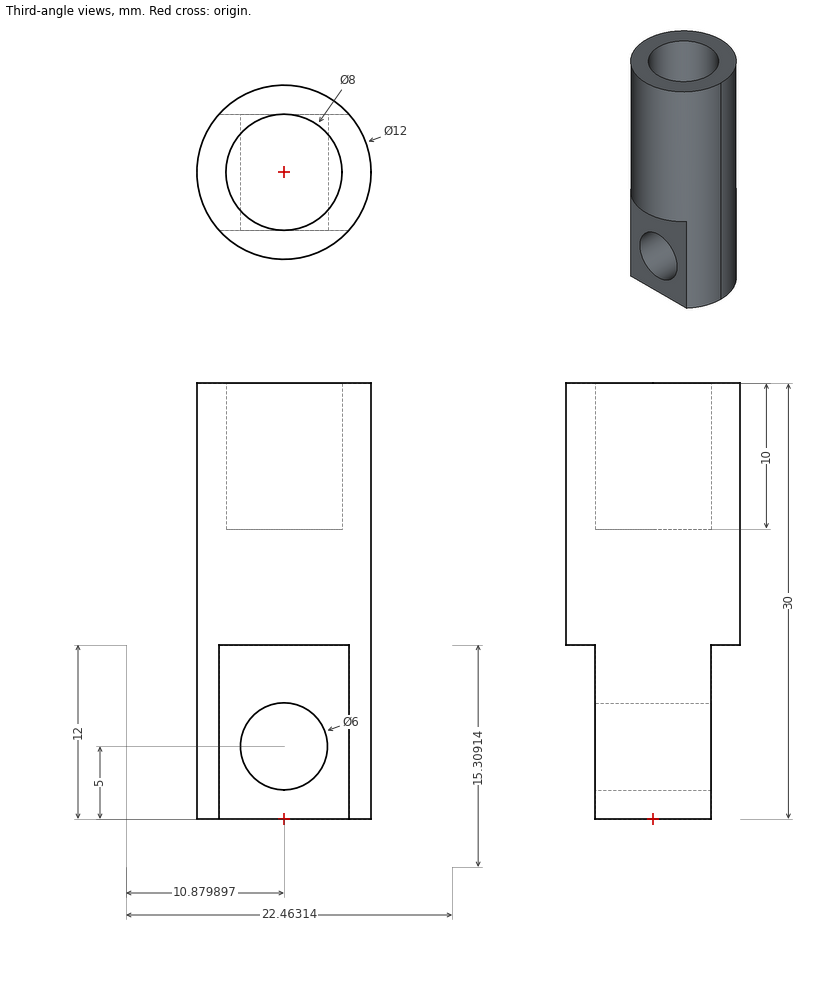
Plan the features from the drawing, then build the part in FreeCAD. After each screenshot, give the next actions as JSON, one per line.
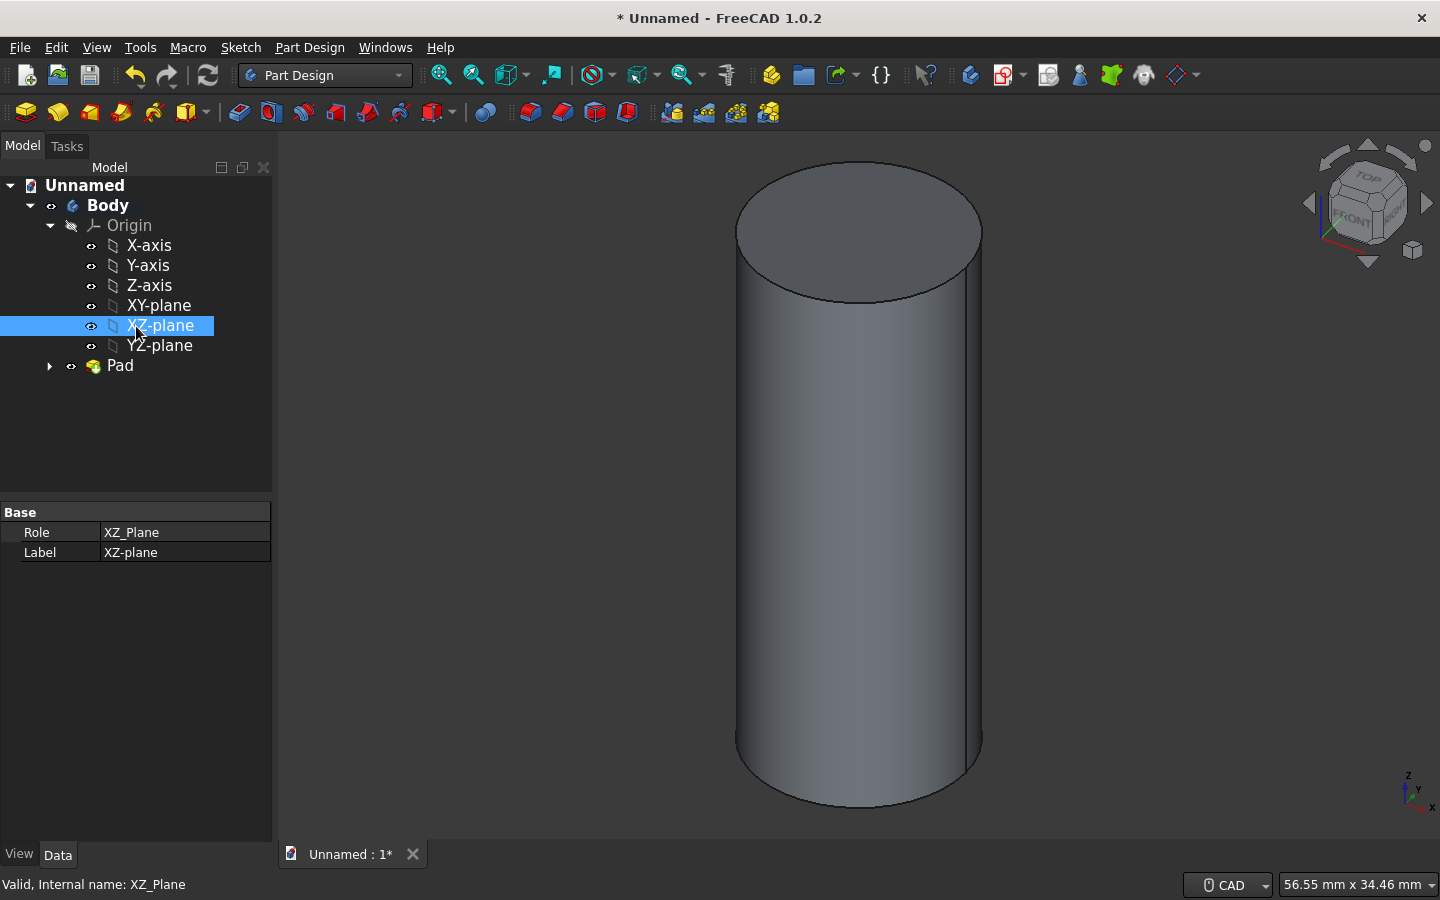
{"action": "left_click", "coordinate": [1176, 76]}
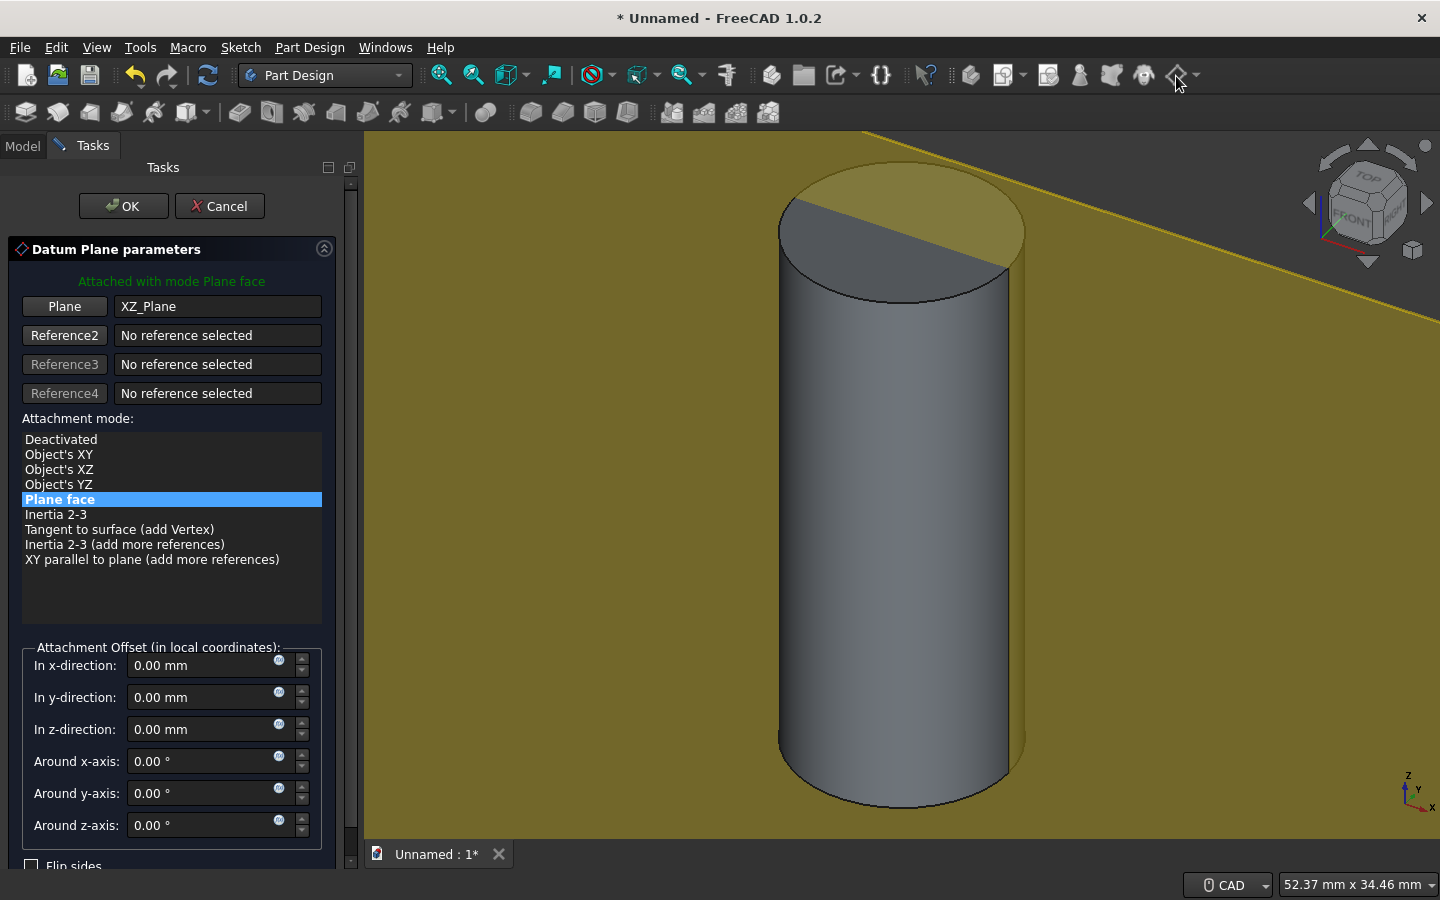
{"action": "triple_click", "coordinate": [210, 729]}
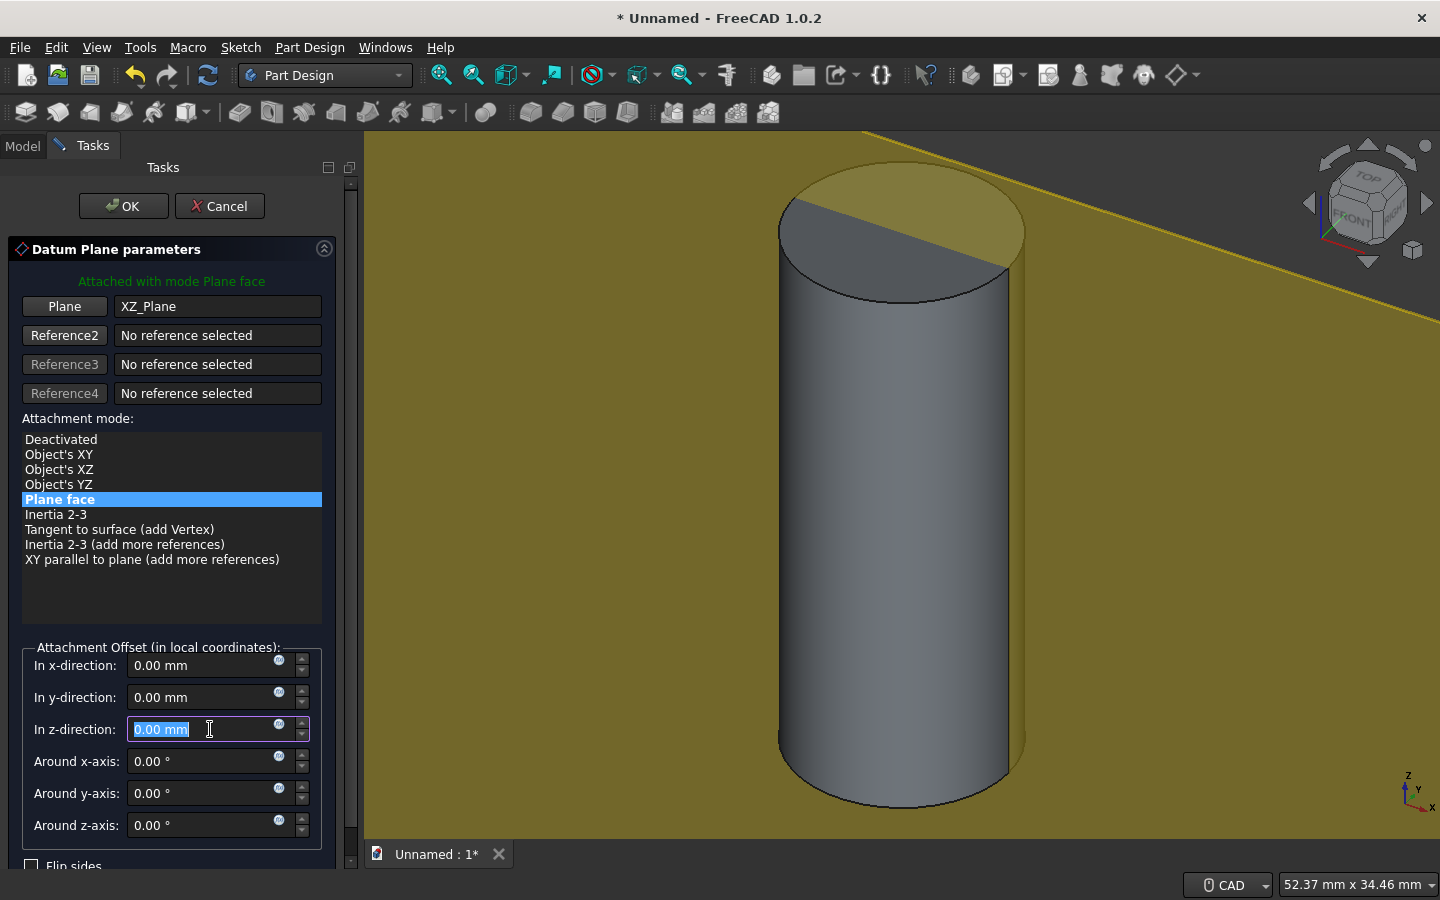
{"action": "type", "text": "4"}
{"action": "key", "text": "Tab"}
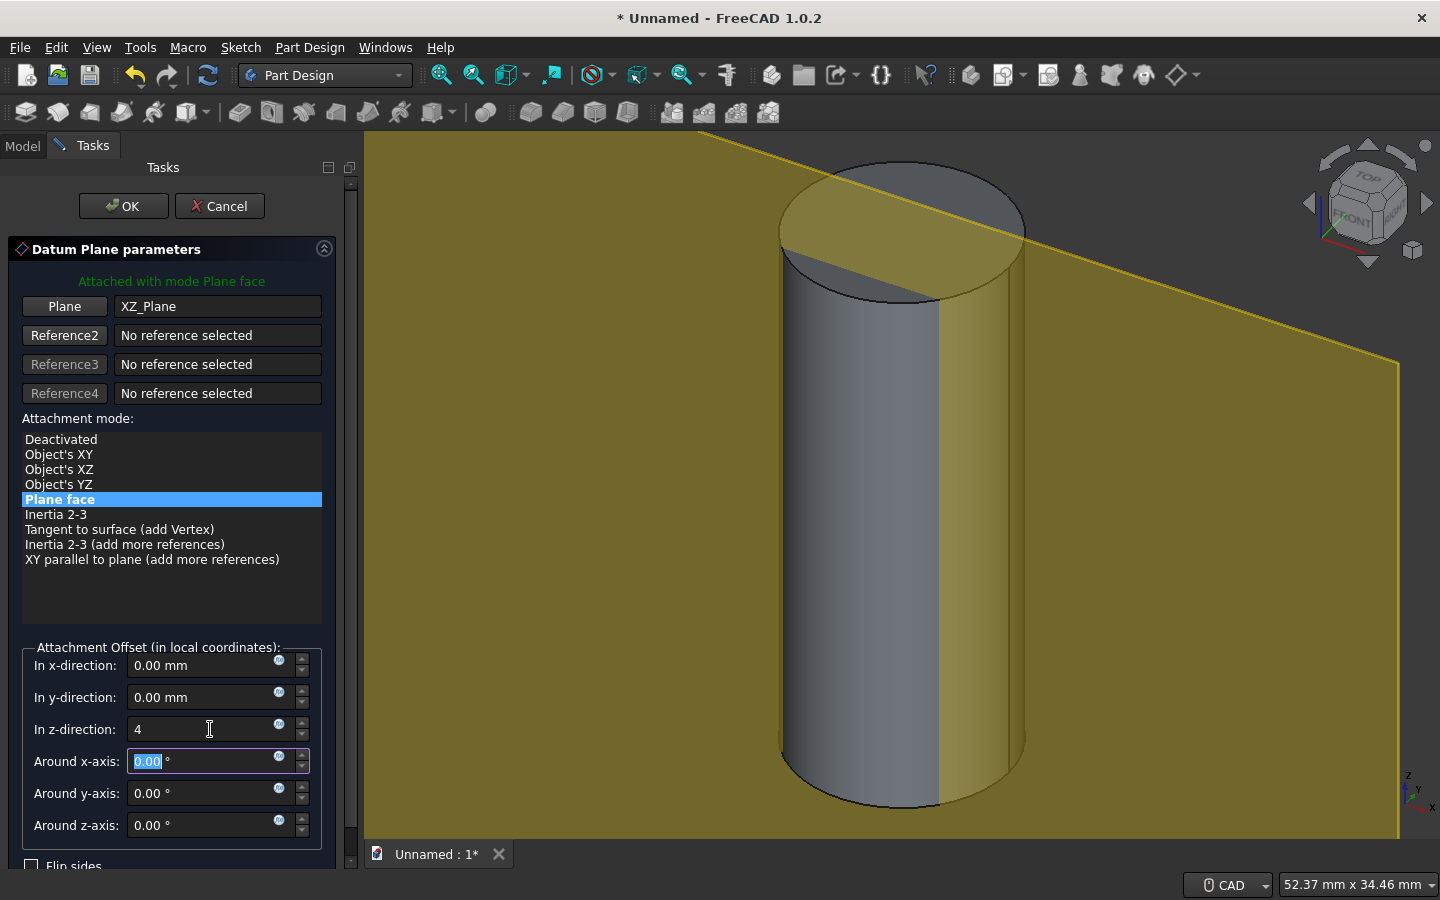
{"action": "left_click", "coordinate": [124, 206]}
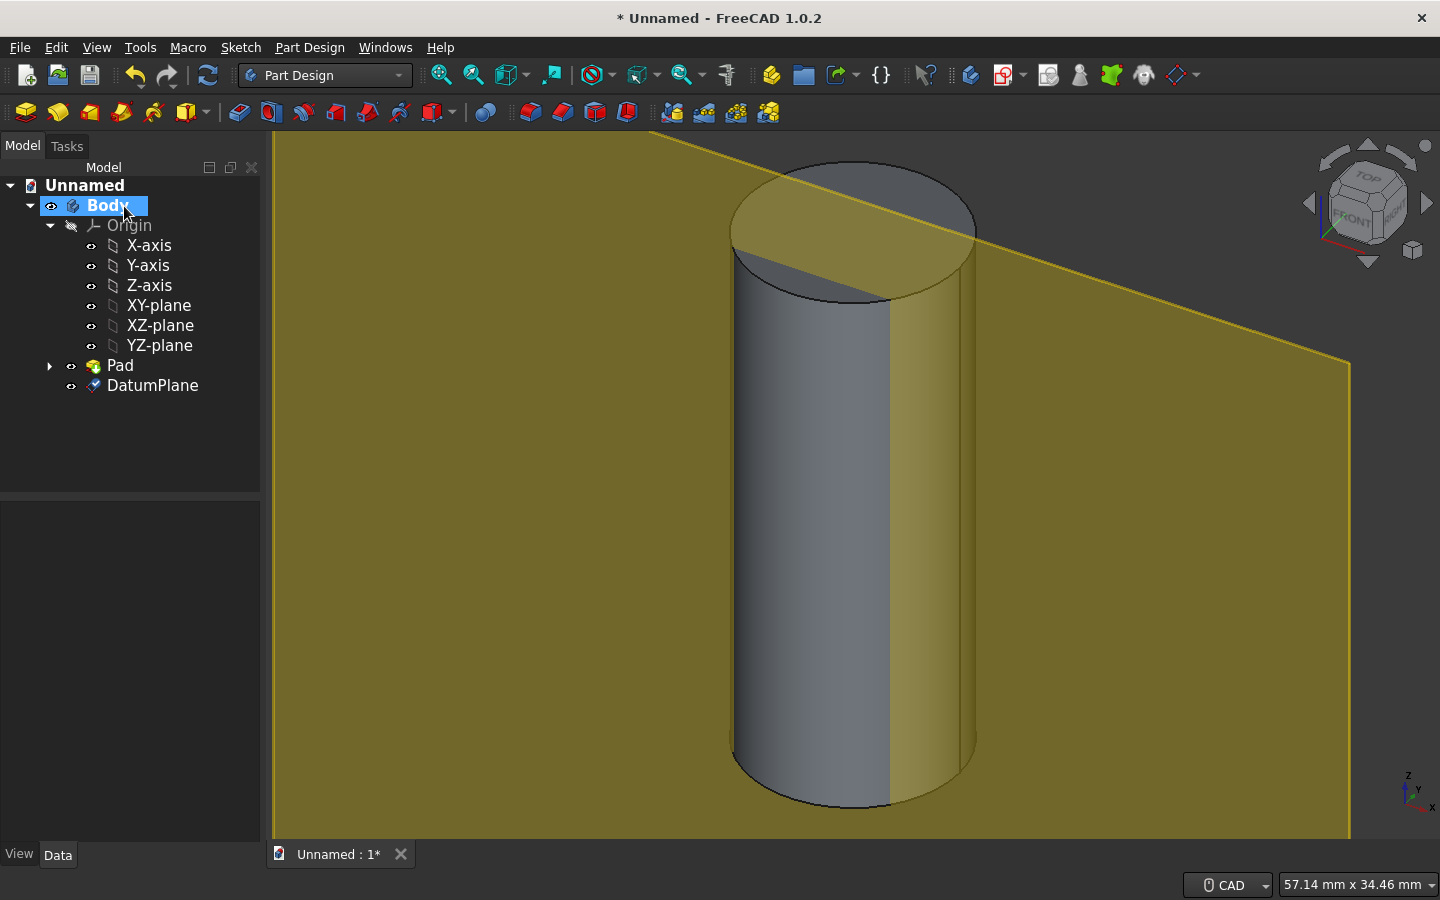
{"action": "left_click", "coordinate": [116, 386]}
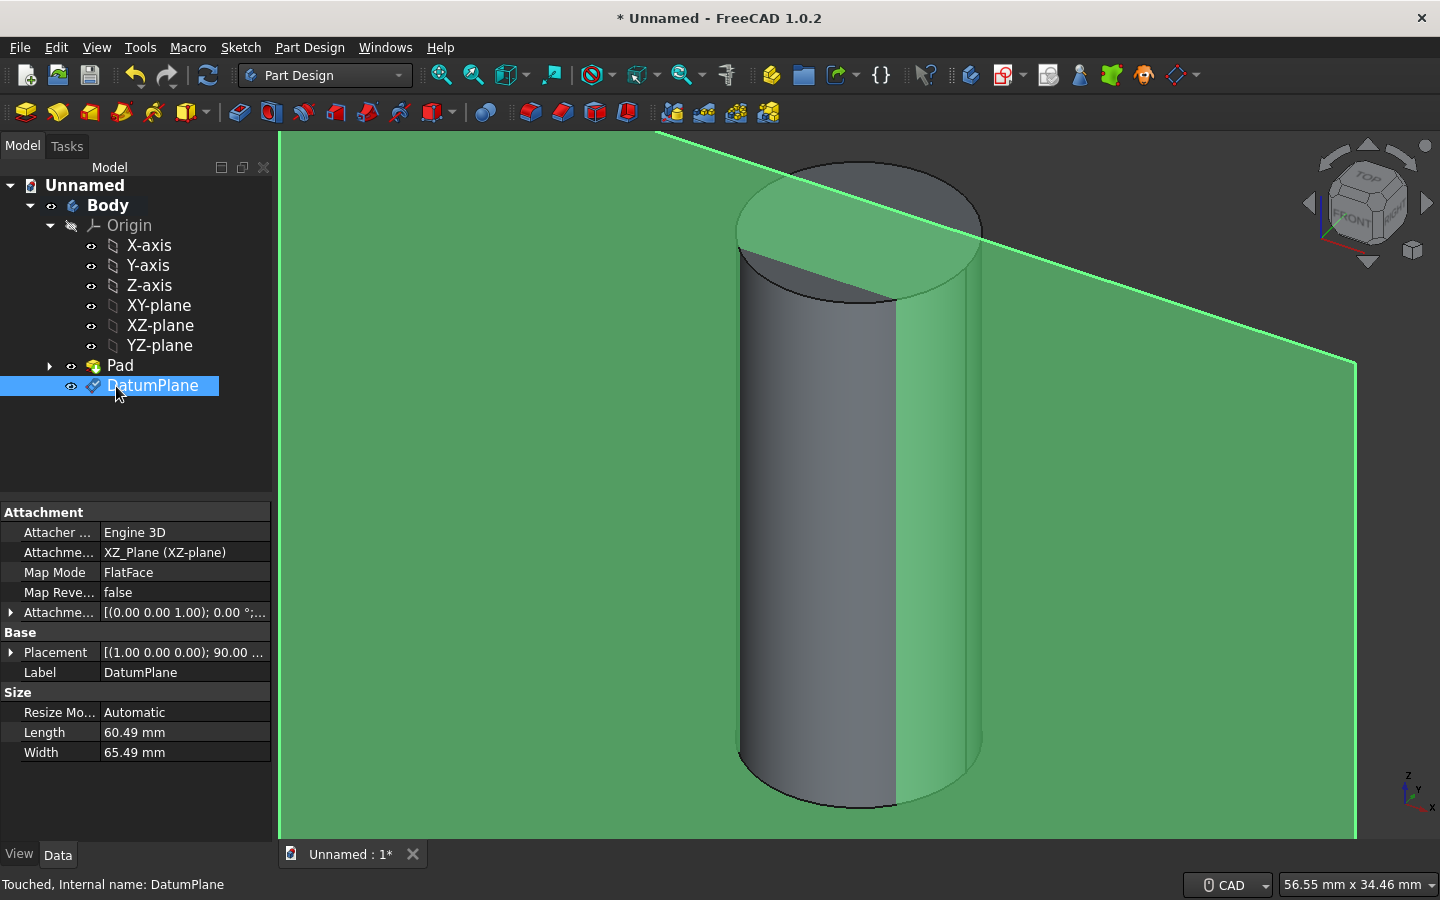
{"action": "left_click", "coordinate": [1004, 76]}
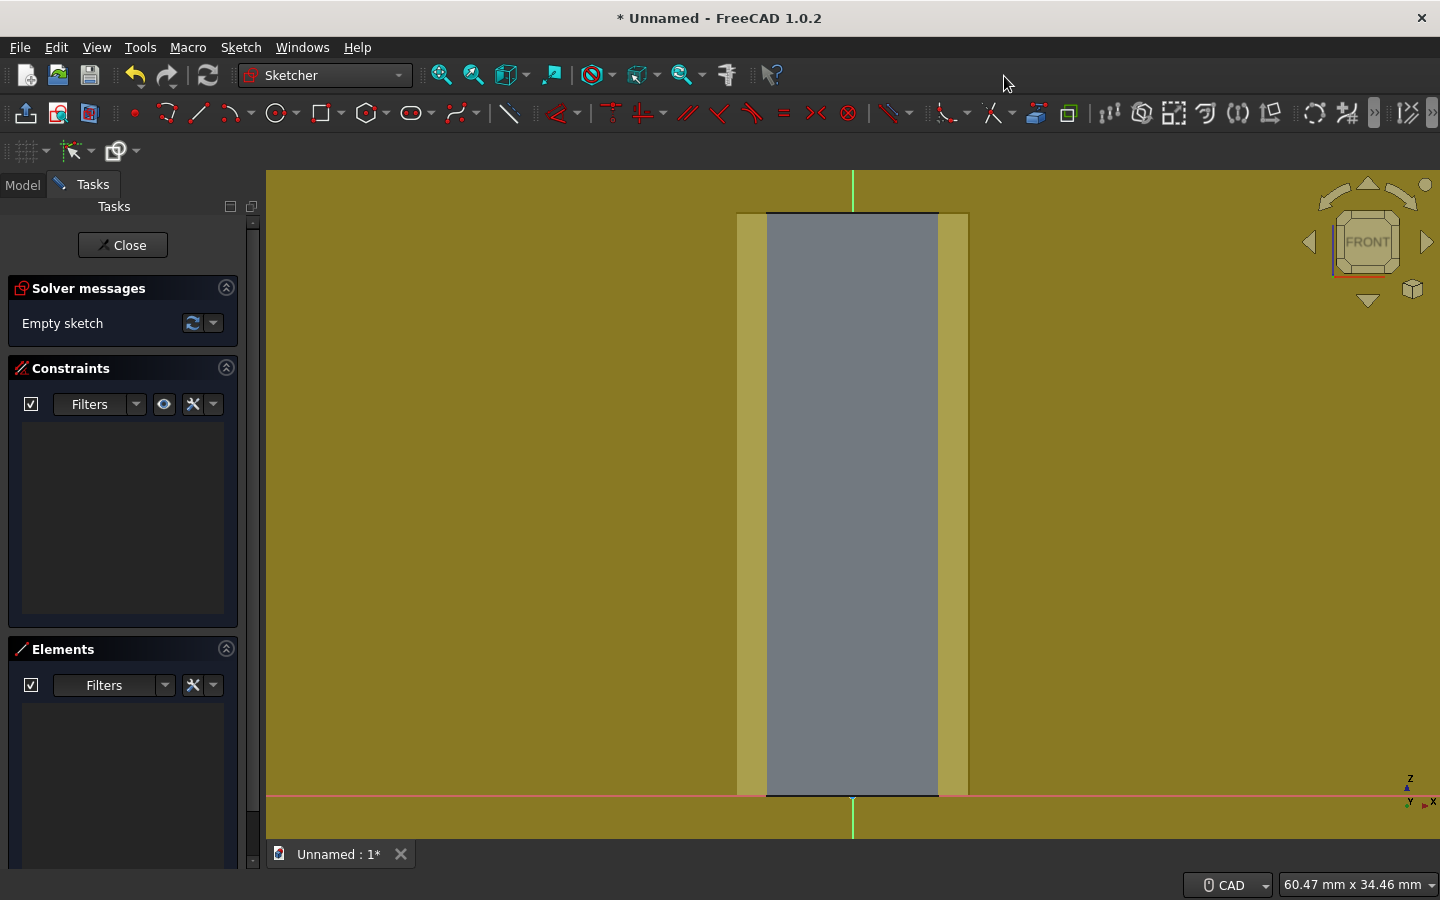
{"action": "left_click", "coordinate": [90, 114]}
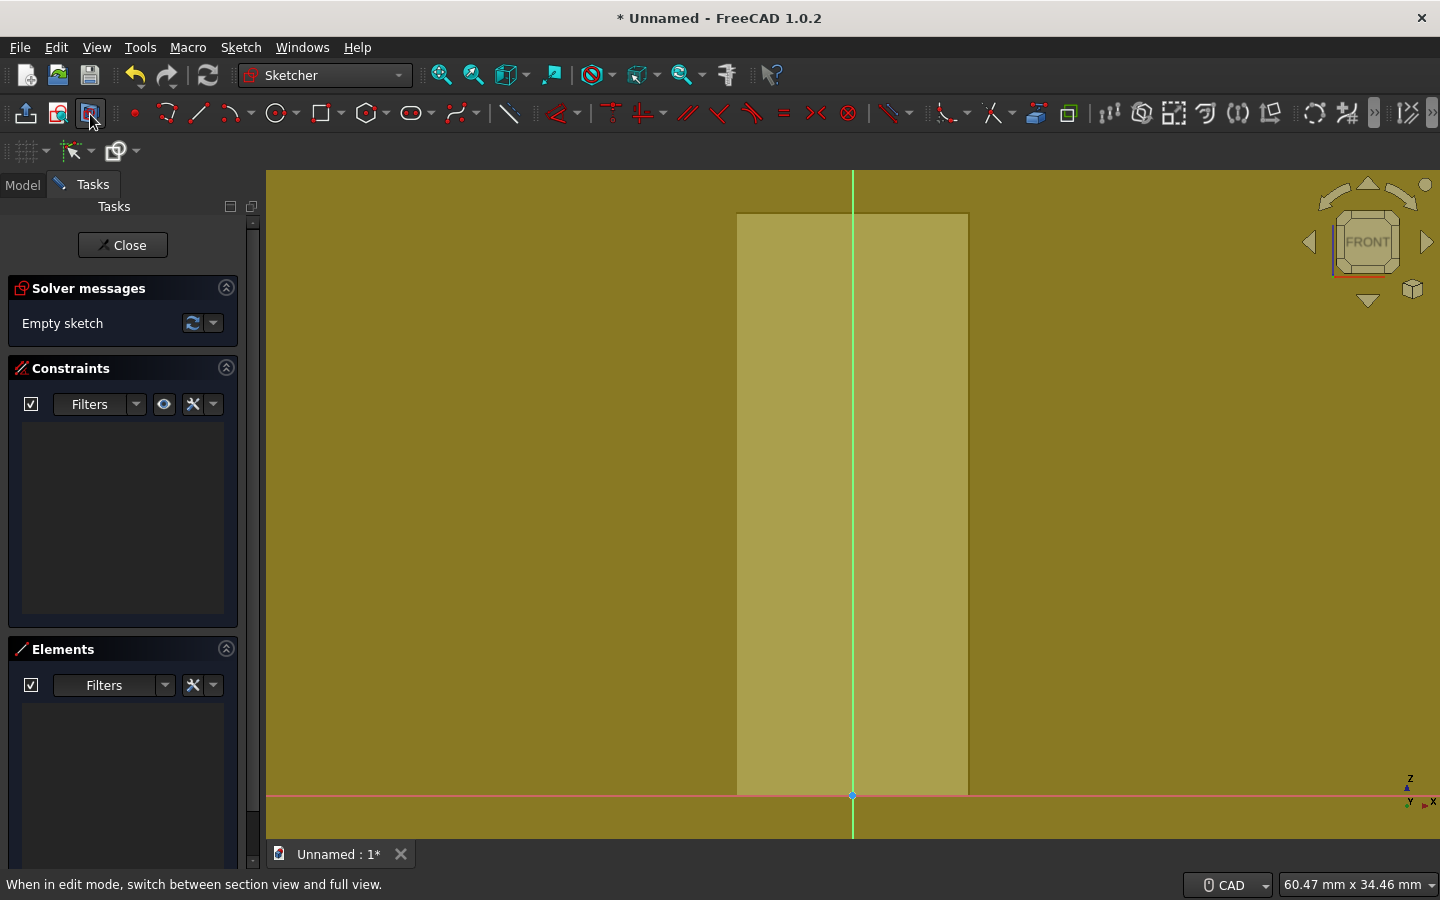
{"action": "scroll", "coordinate": [445, 198], "scroll_direction": "down", "scroll_amount": 1}